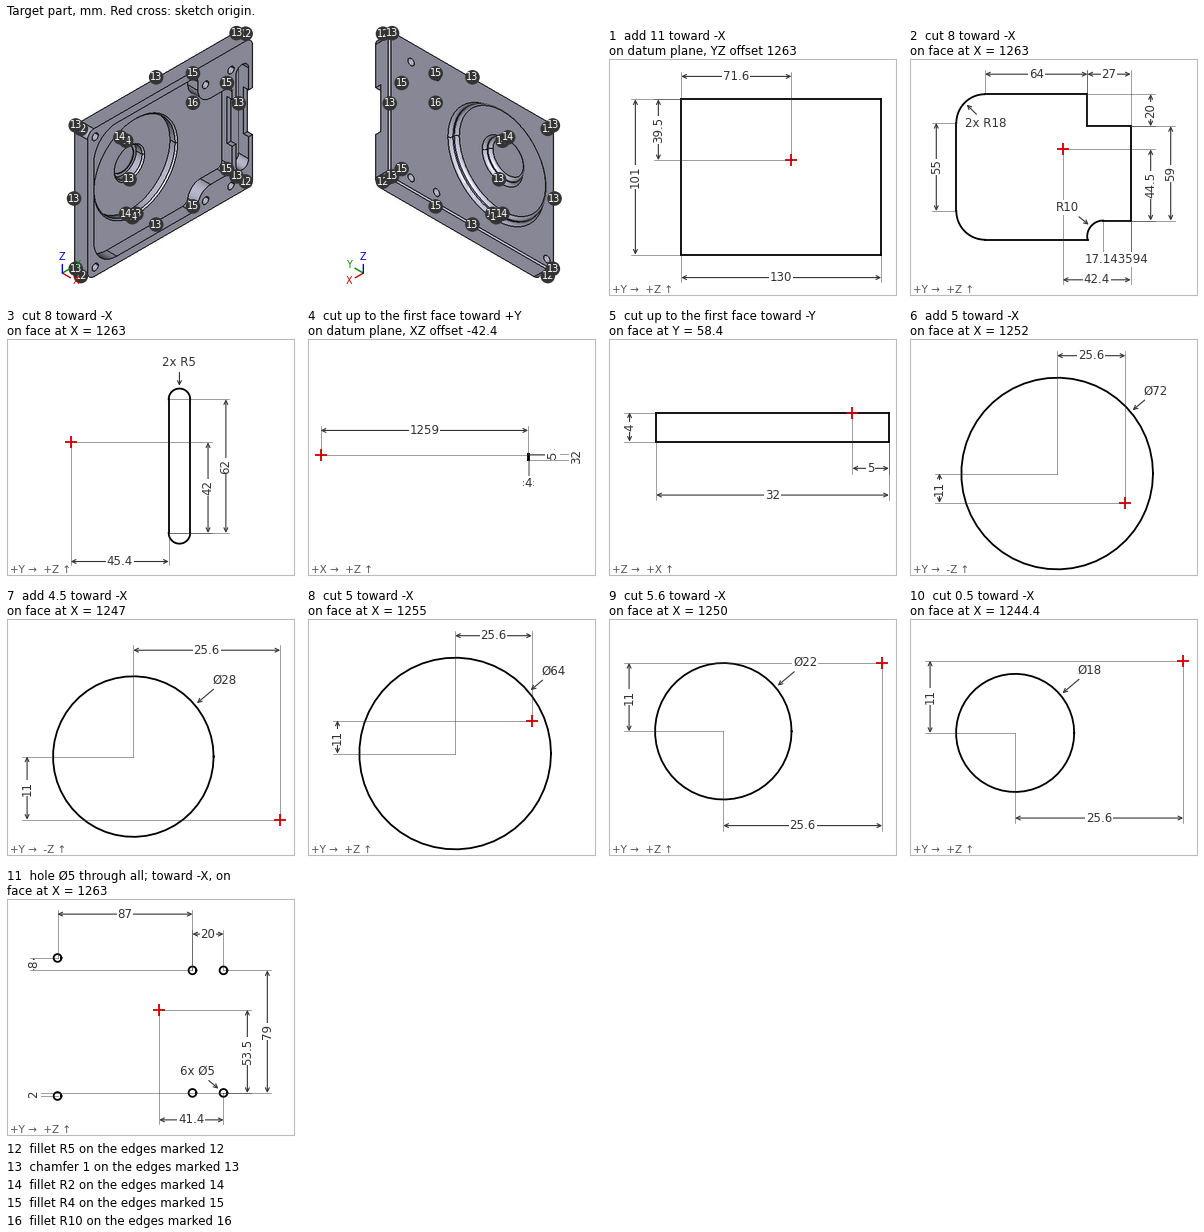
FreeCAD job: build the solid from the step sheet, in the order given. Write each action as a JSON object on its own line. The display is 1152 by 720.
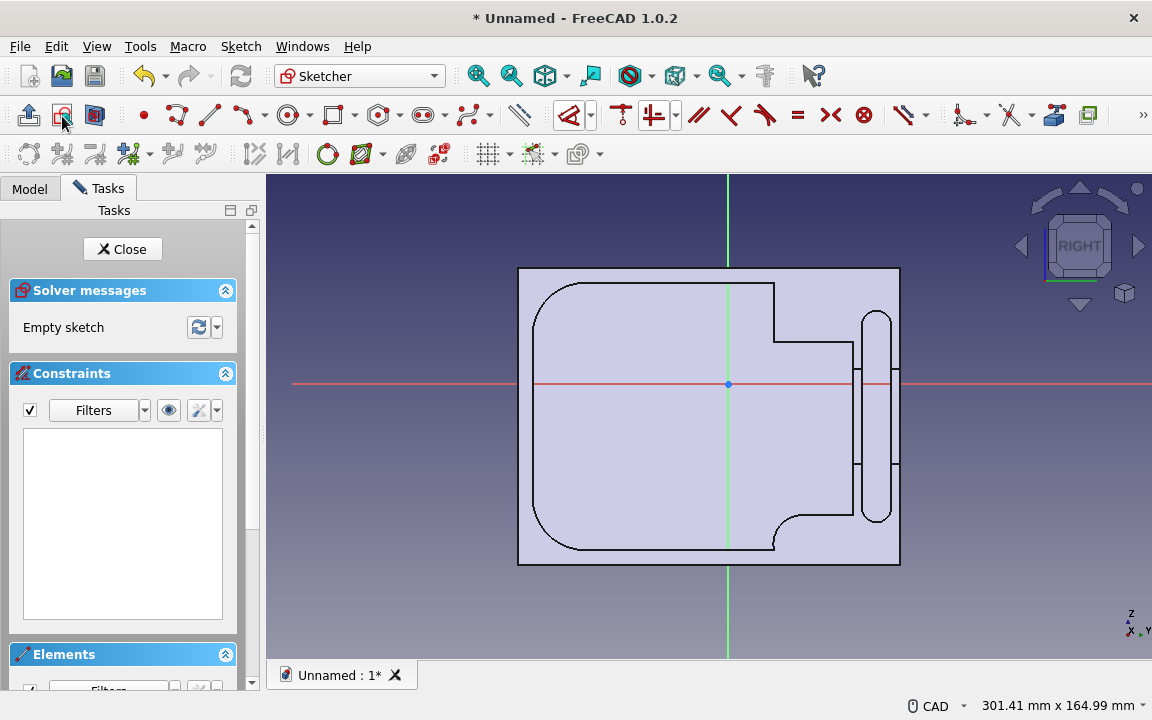
{"action": "left_click", "coordinate": [95, 116]}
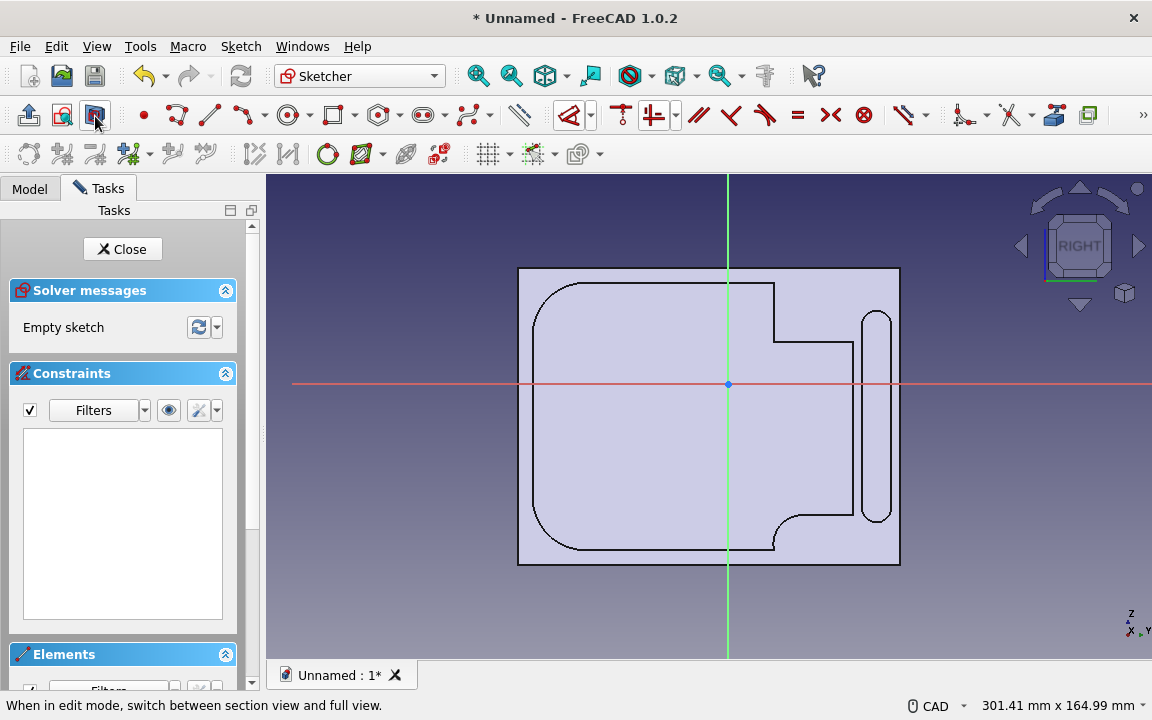
{"action": "scroll", "coordinate": [679, 417], "scroll_direction": "up", "scroll_amount": 2}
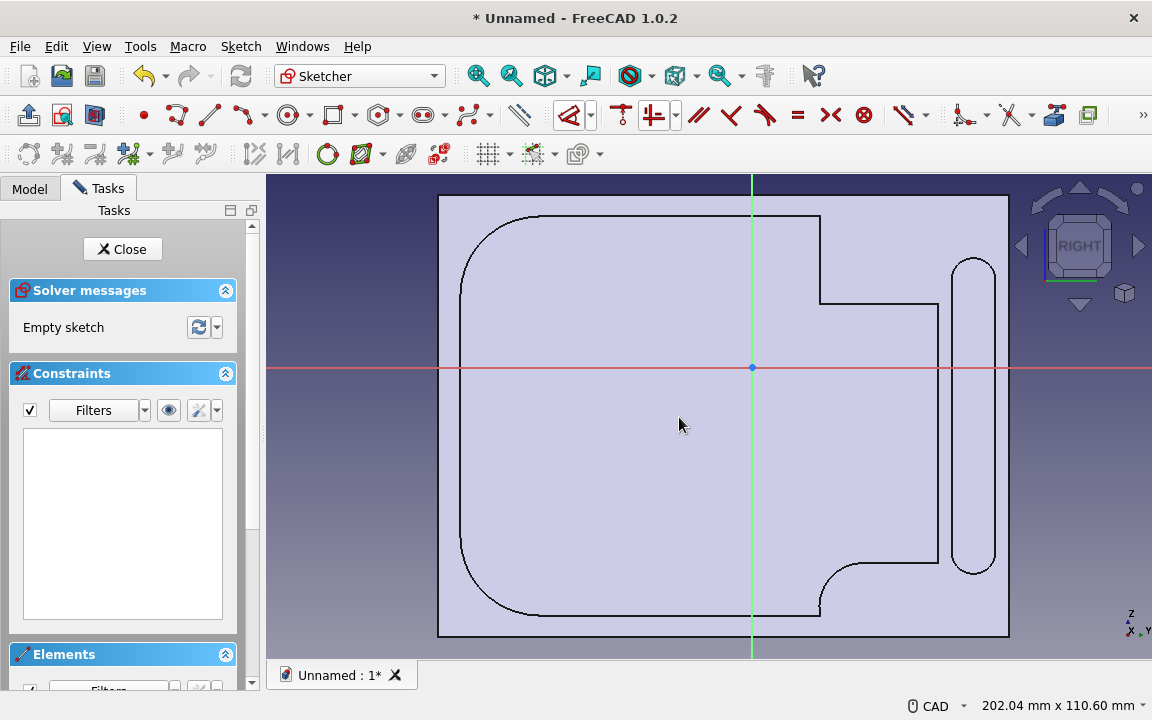
{"action": "left_click", "coordinate": [288, 116]}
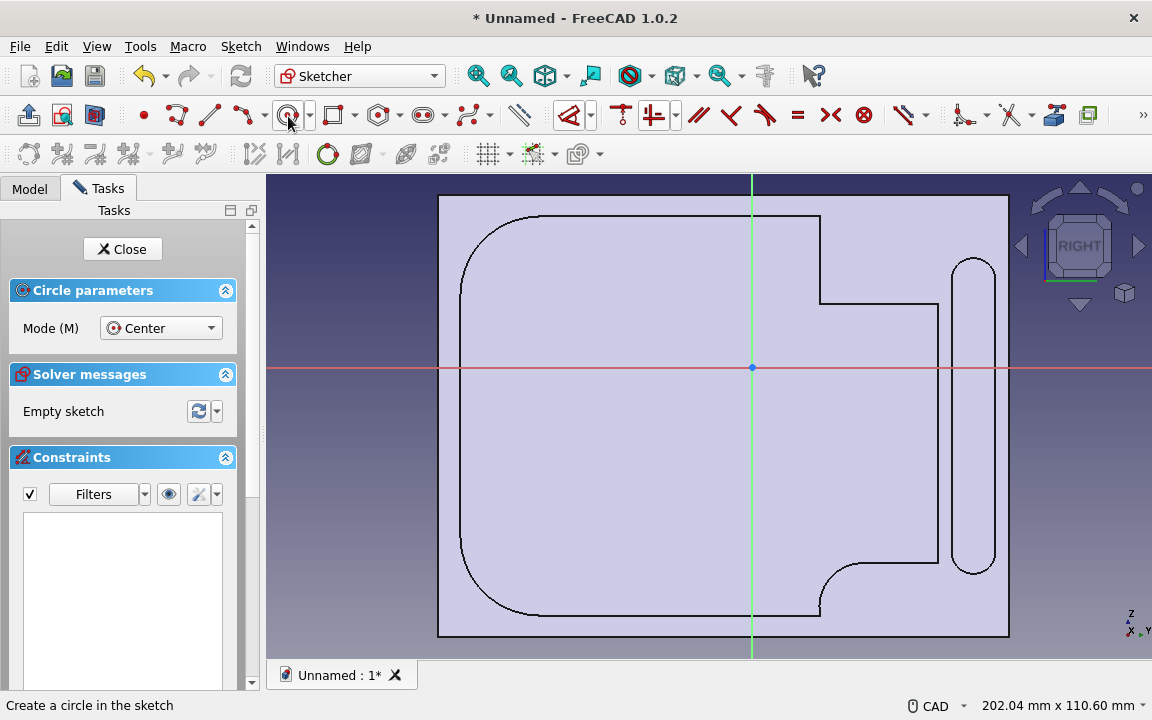
{"action": "left_click", "coordinate": [640, 416]}
{"action": "left_click", "coordinate": [541, 317]}
{"action": "key", "text": "Escape"}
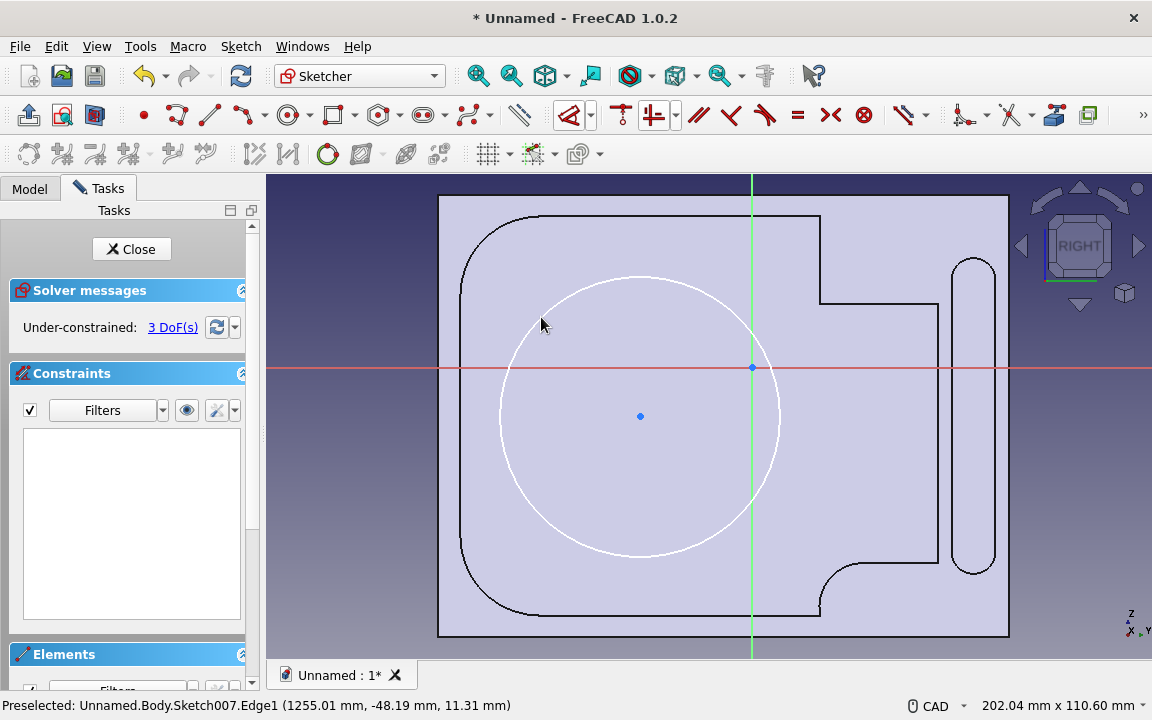
{"action": "left_click", "coordinate": [739, 318]}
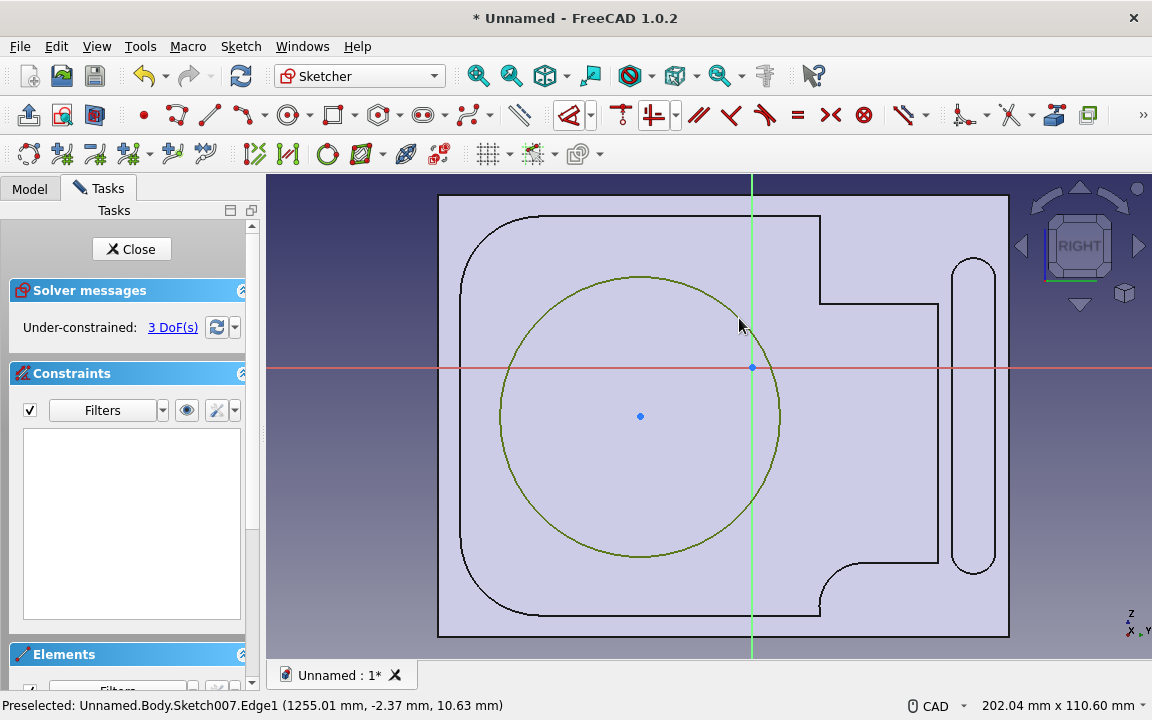
{"action": "left_click", "coordinate": [590, 116]}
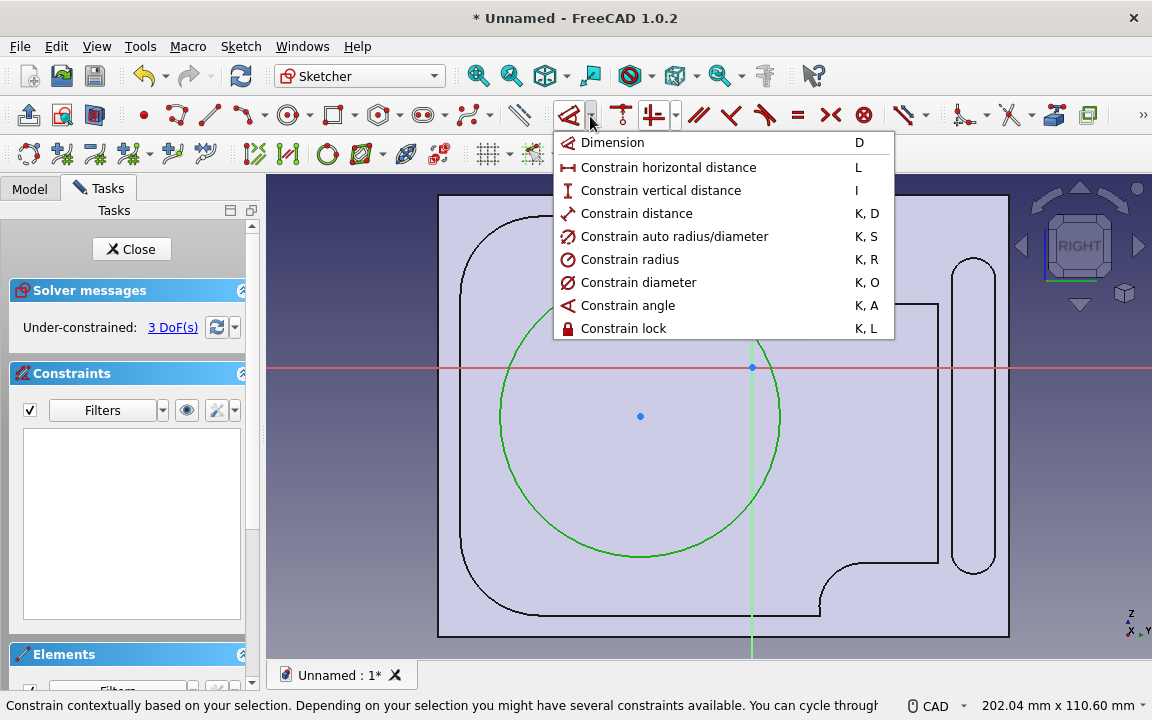
{"action": "left_click", "coordinate": [724, 282]}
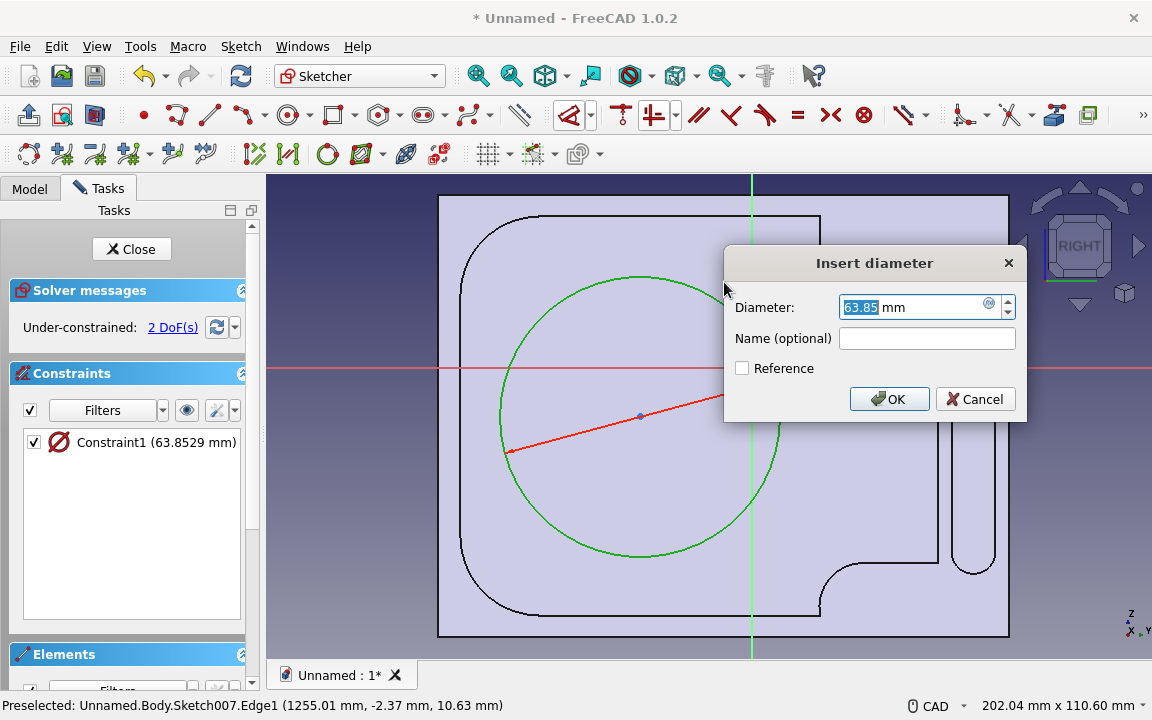
{"action": "type", "text": "64"}
{"action": "key", "text": "Return"}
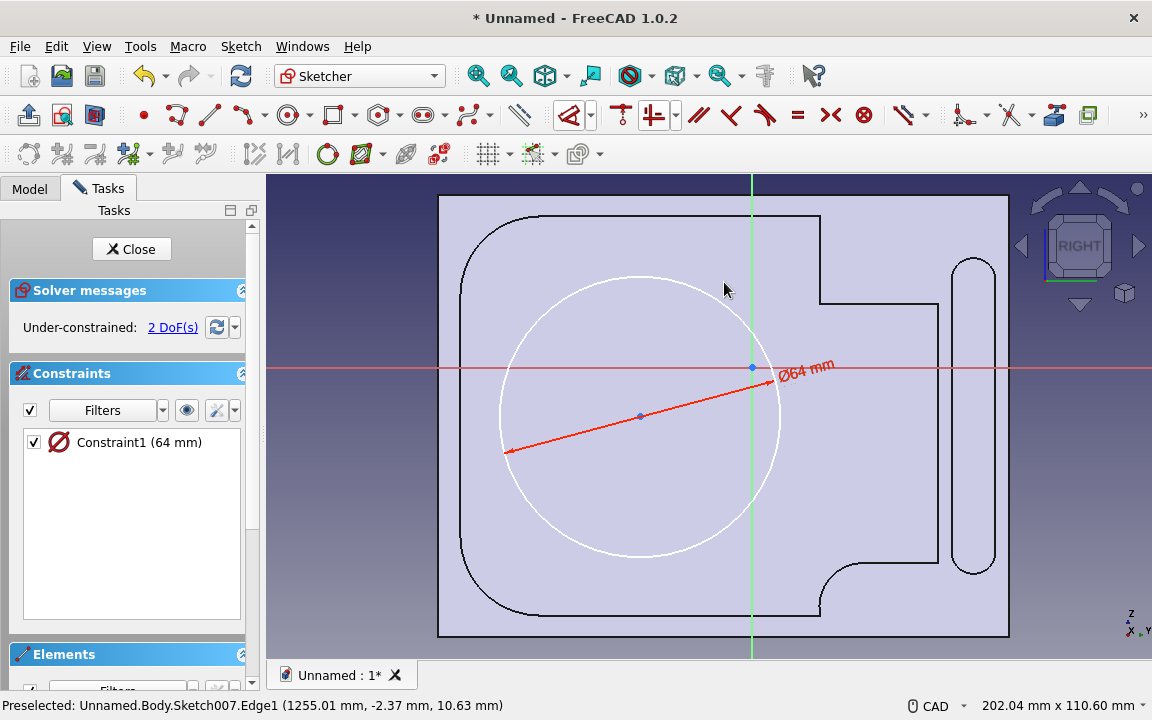
{"action": "left_click", "coordinate": [640, 417]}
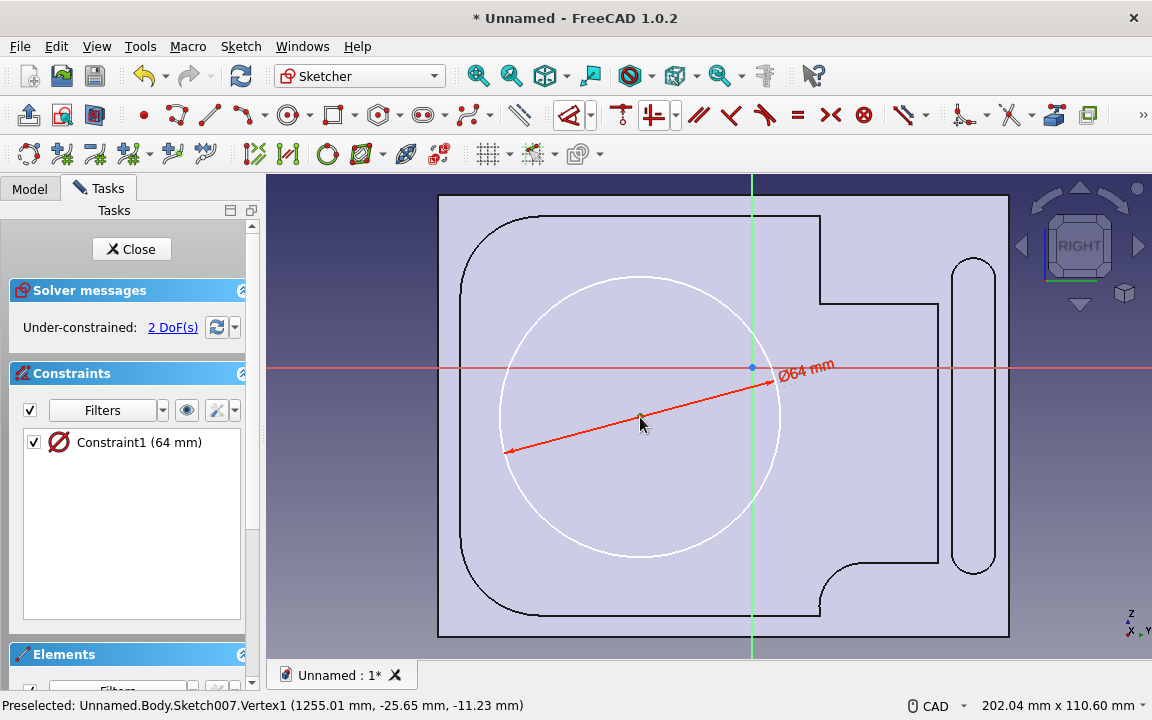
{"action": "left_click", "coordinate": [590, 116]}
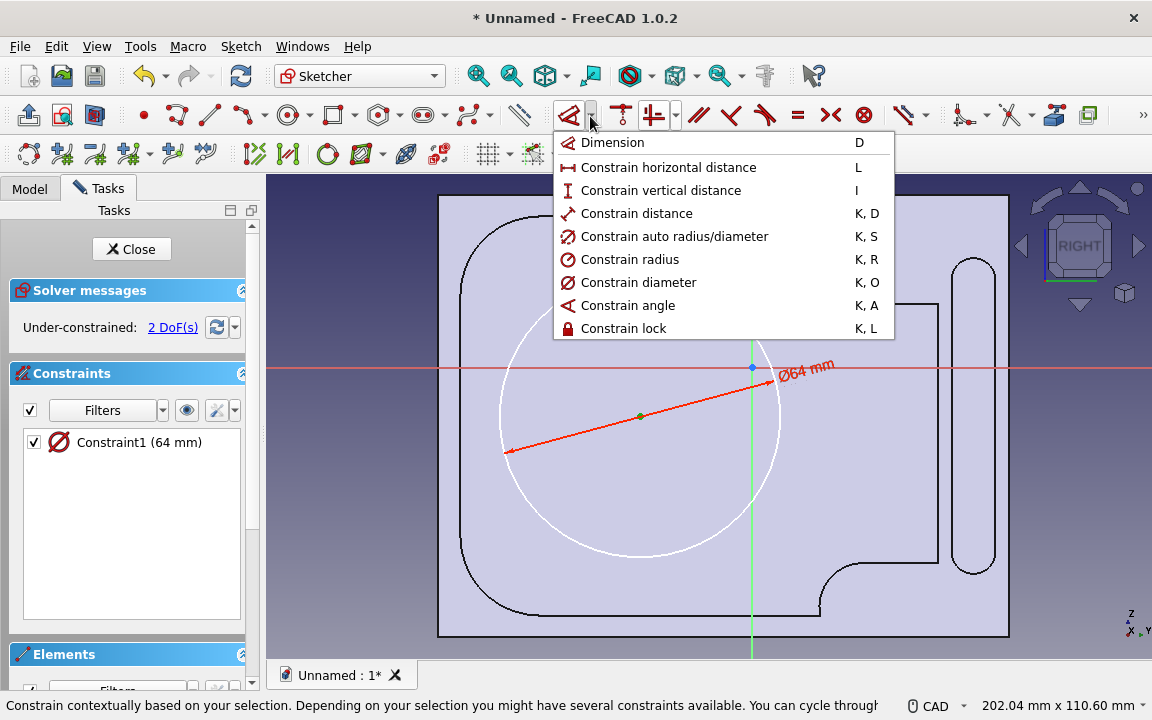
{"action": "left_click", "coordinate": [724, 190]}